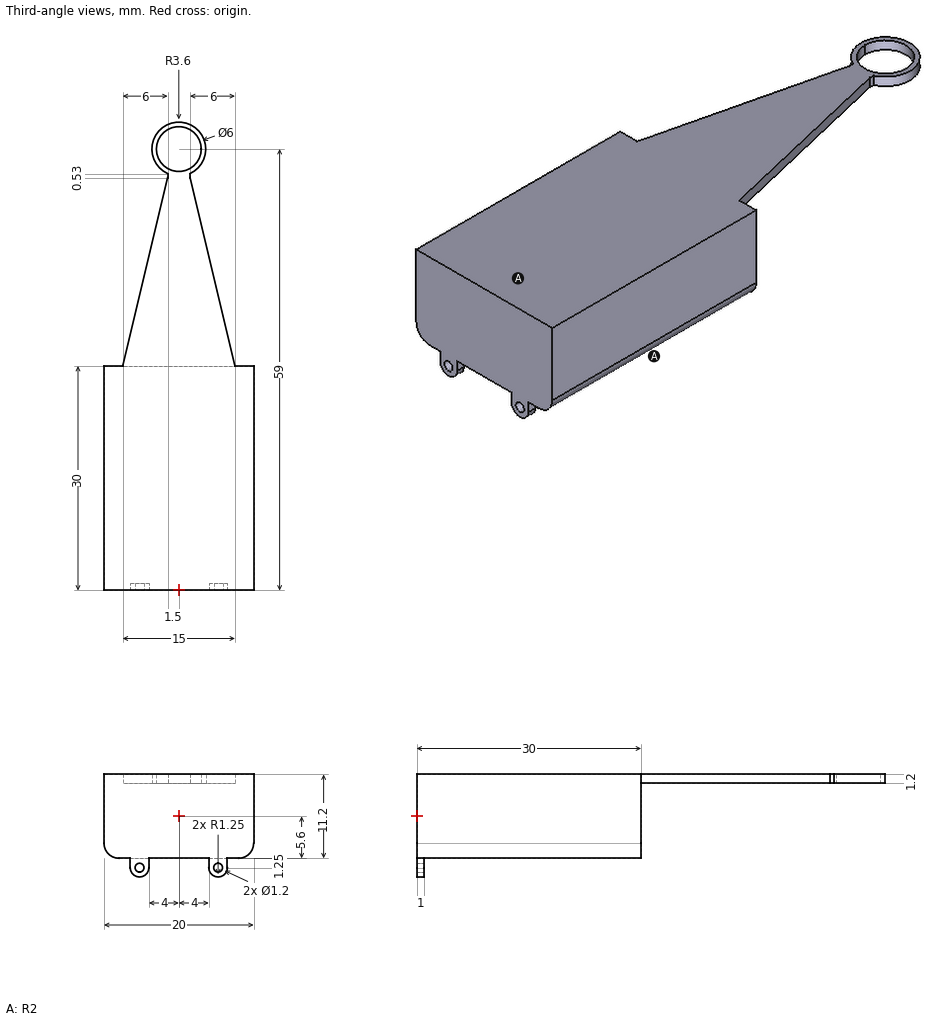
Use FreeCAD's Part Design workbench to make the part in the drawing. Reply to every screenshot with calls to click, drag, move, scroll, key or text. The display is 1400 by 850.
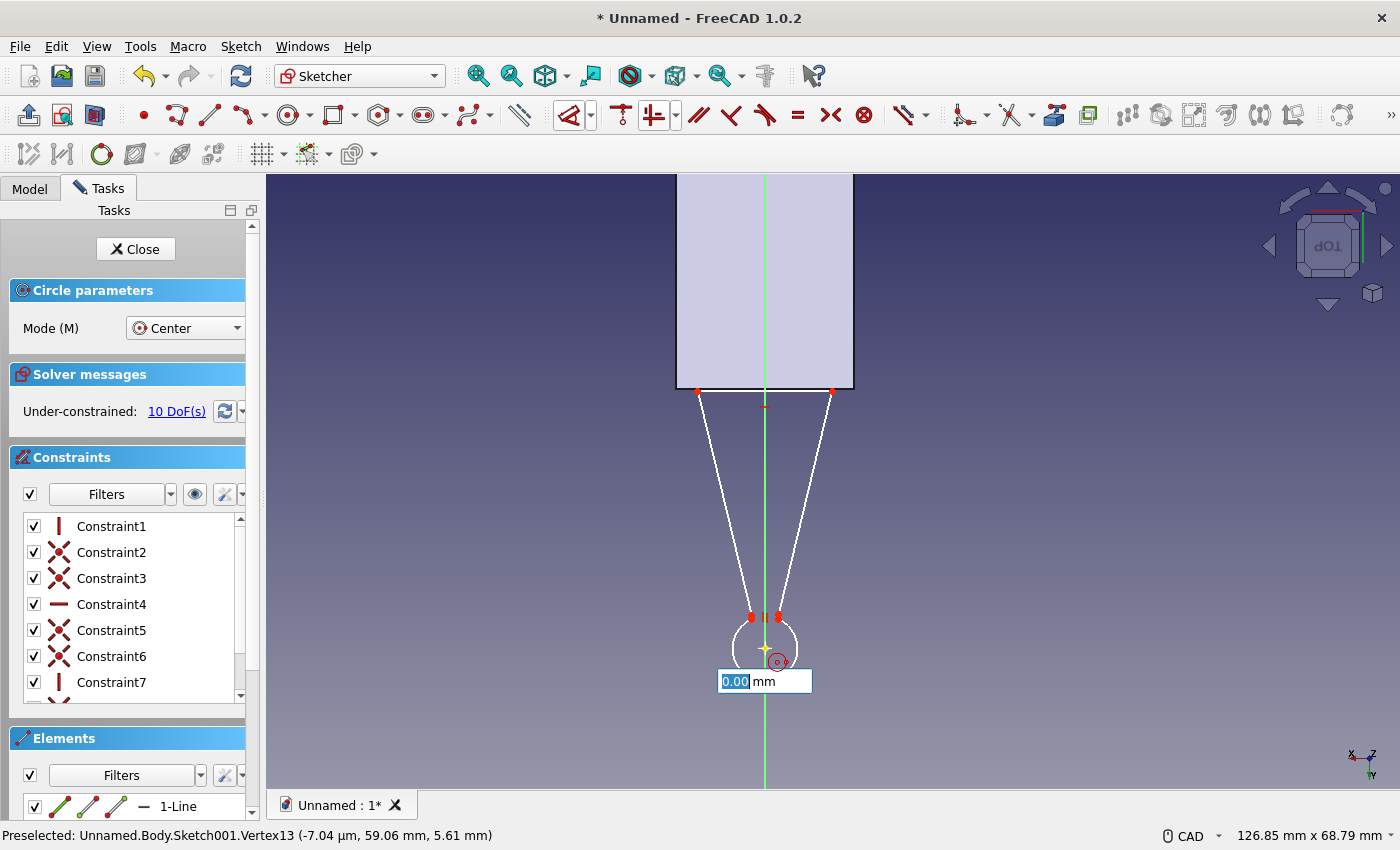
scroll(774, 623, up, 5)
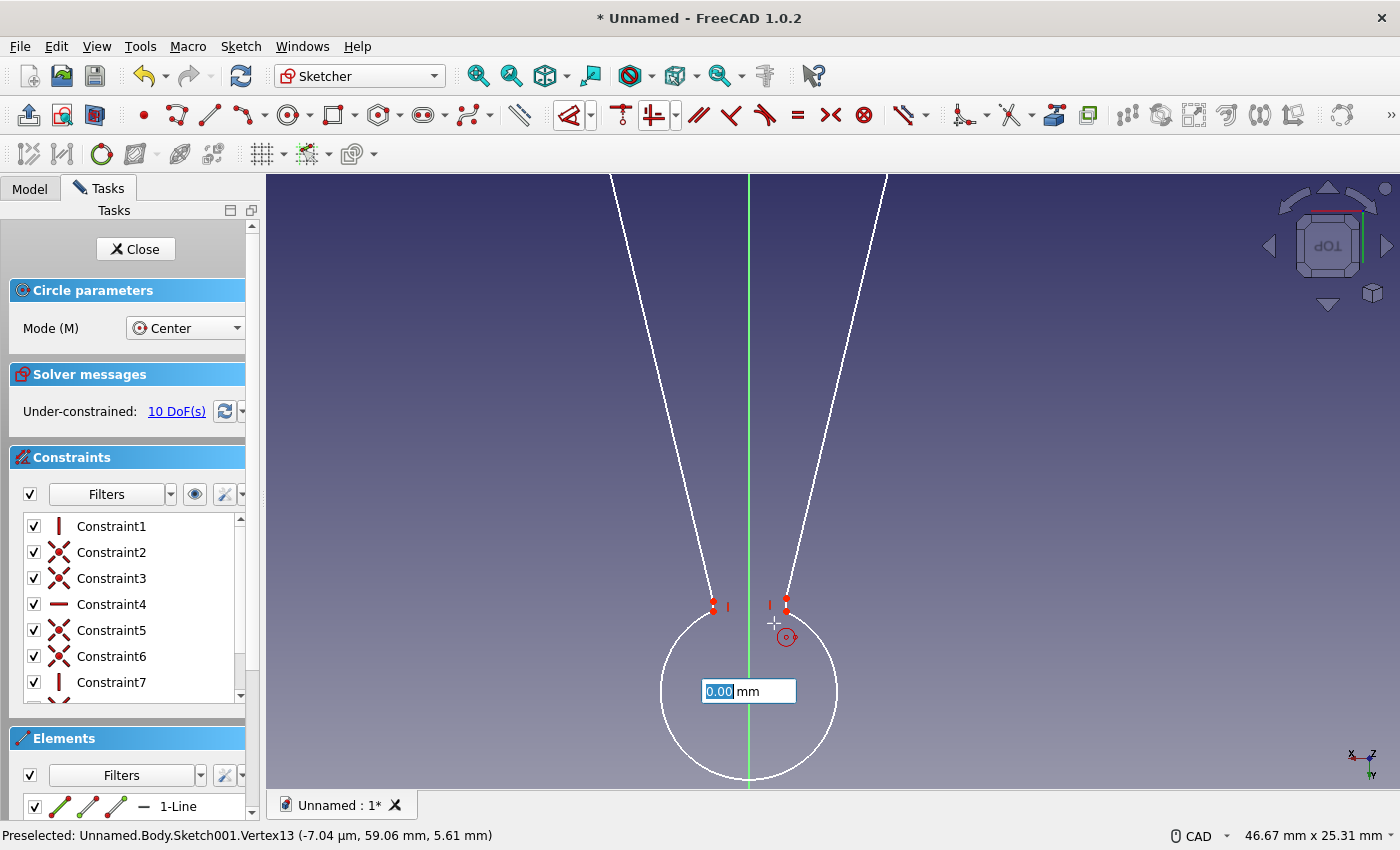
click(774, 622)
key(Escape)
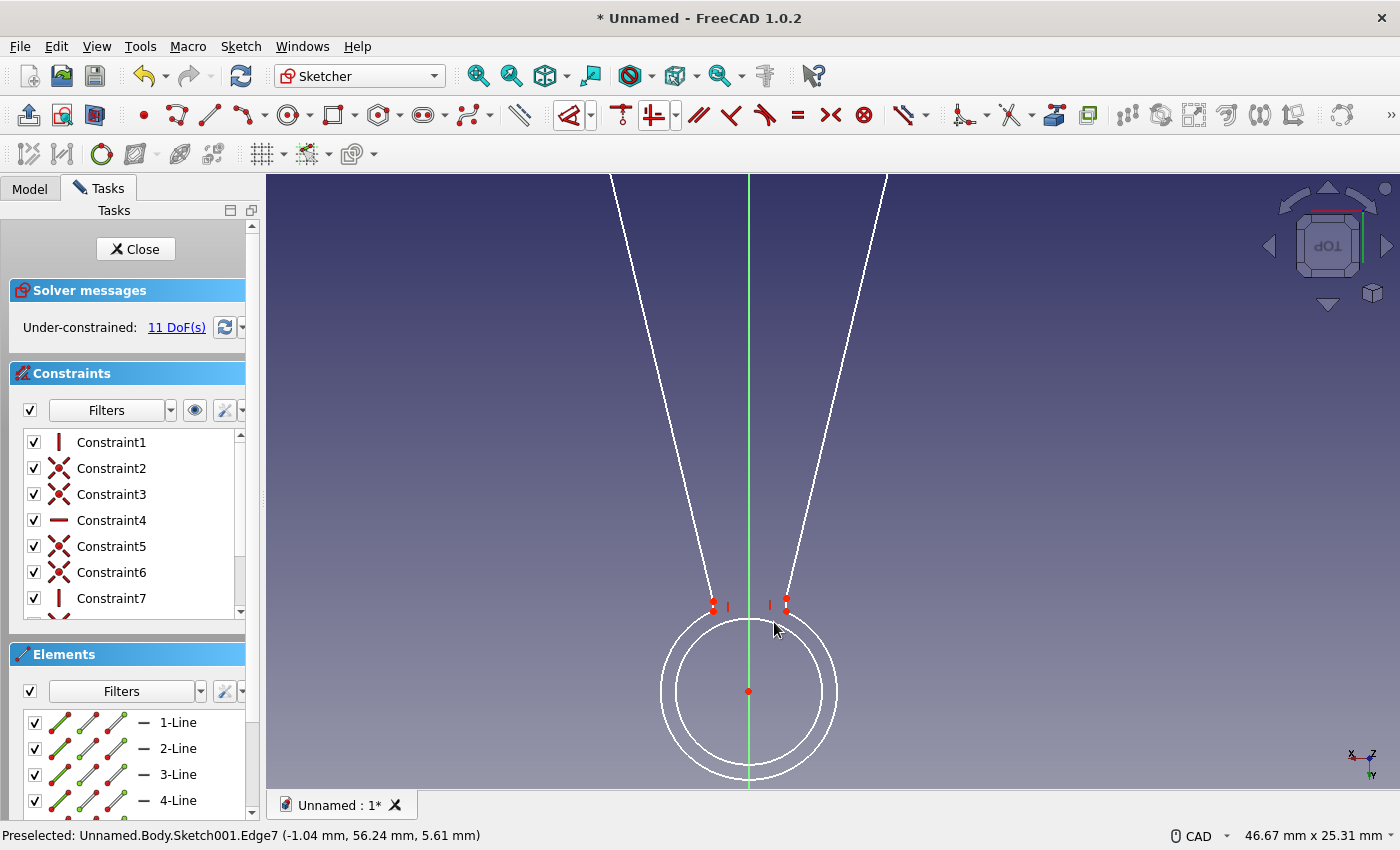
scroll(770, 634, down, 7)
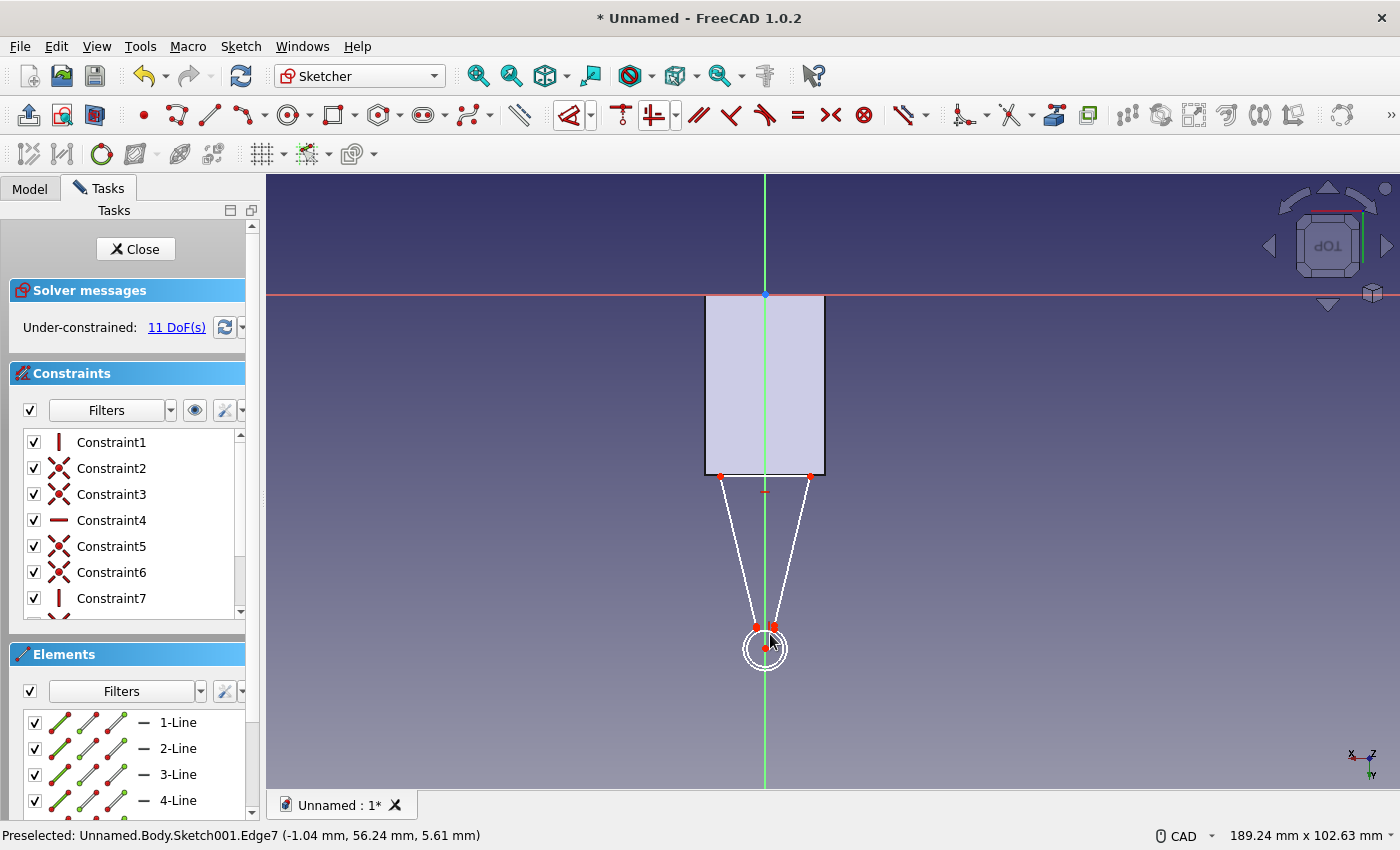
click(765, 649)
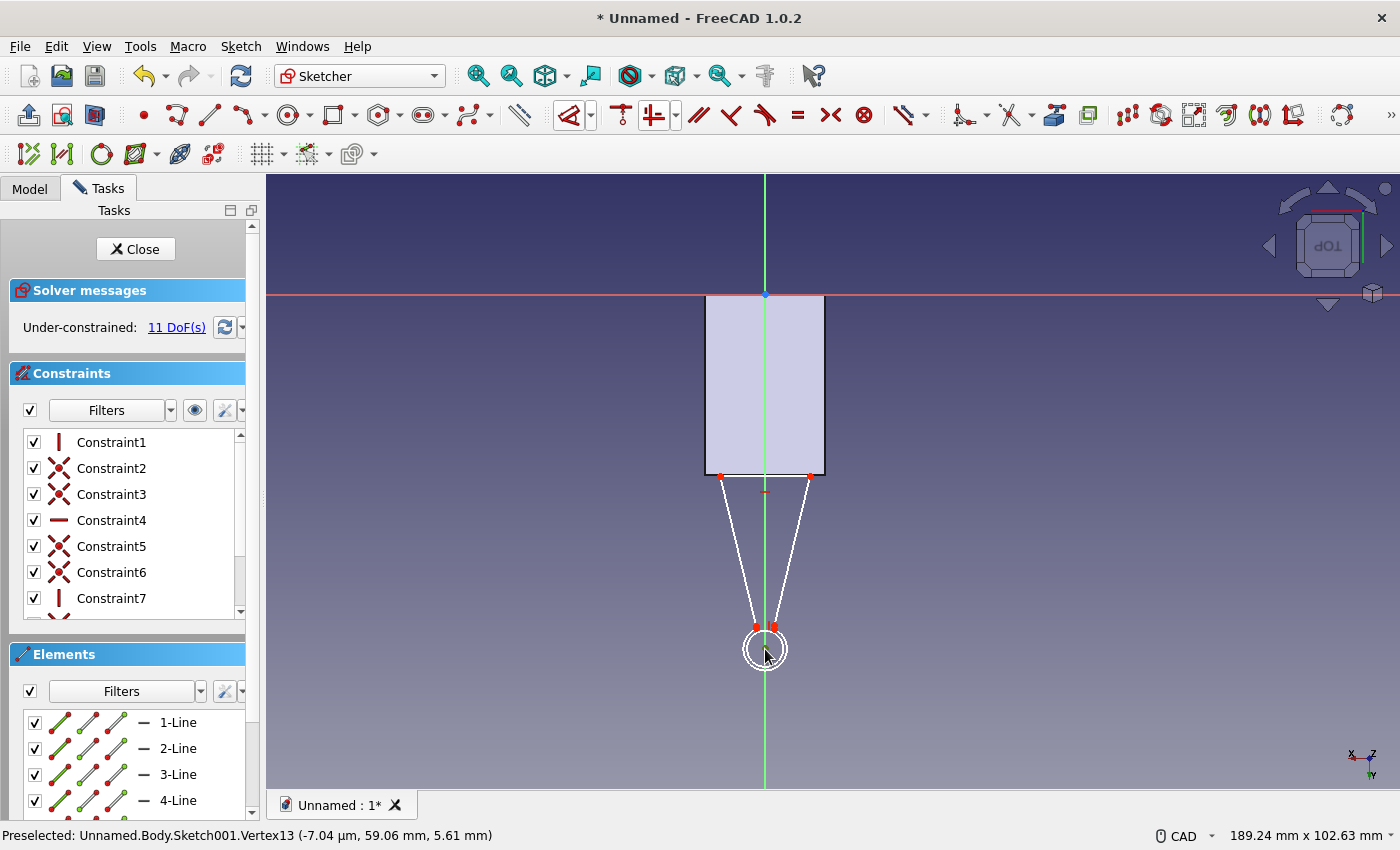
click(765, 721)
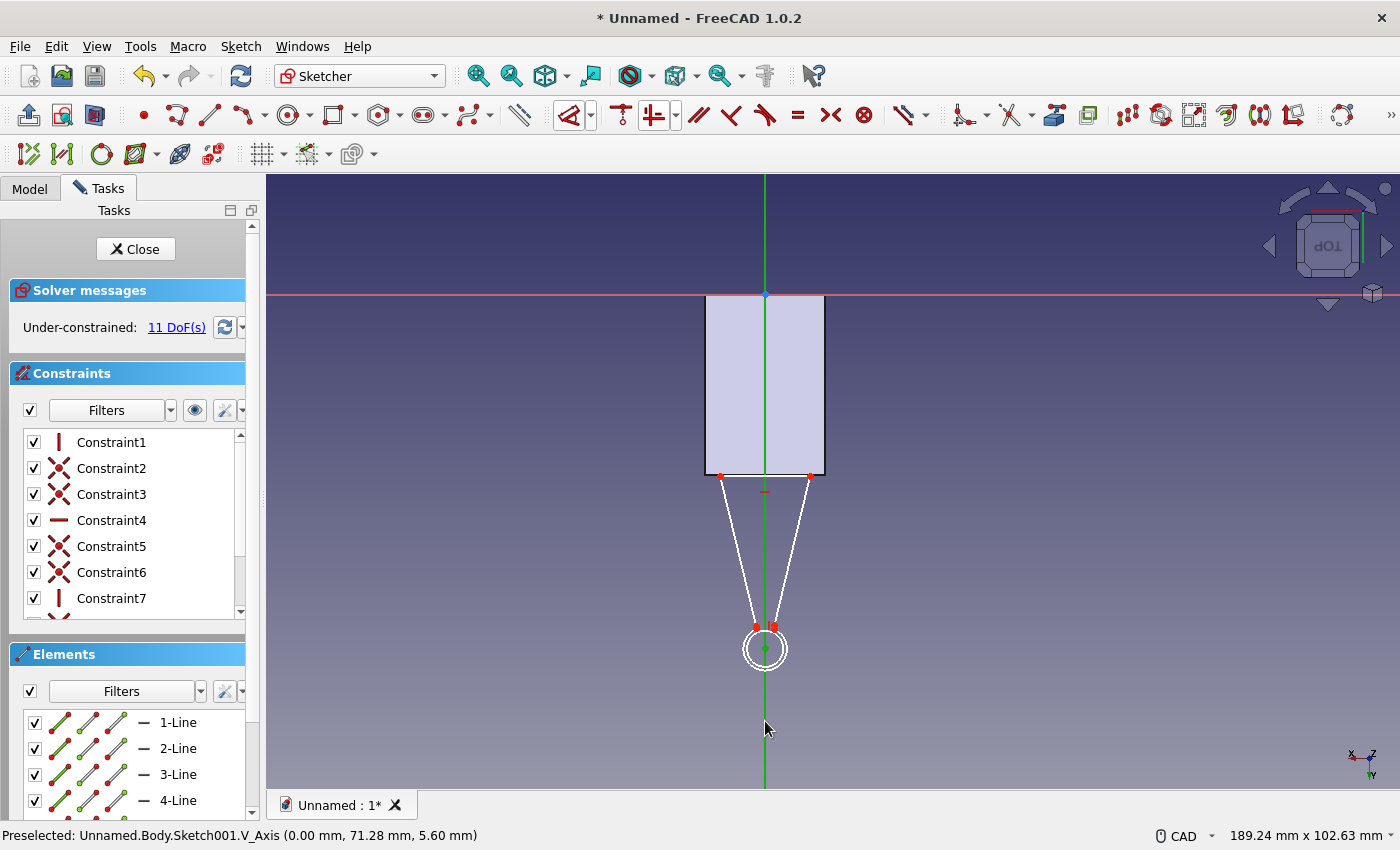
key(c)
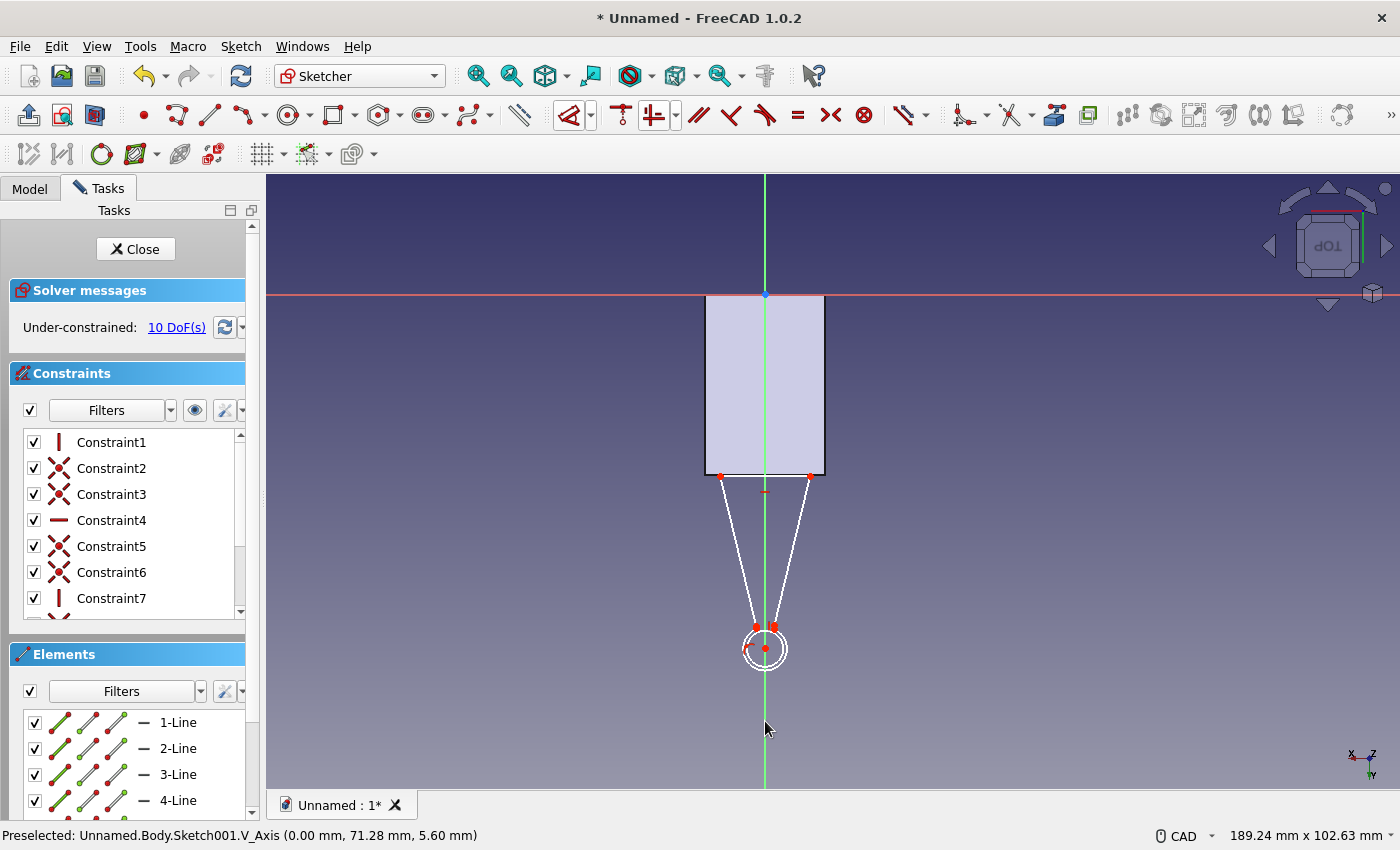
key(d)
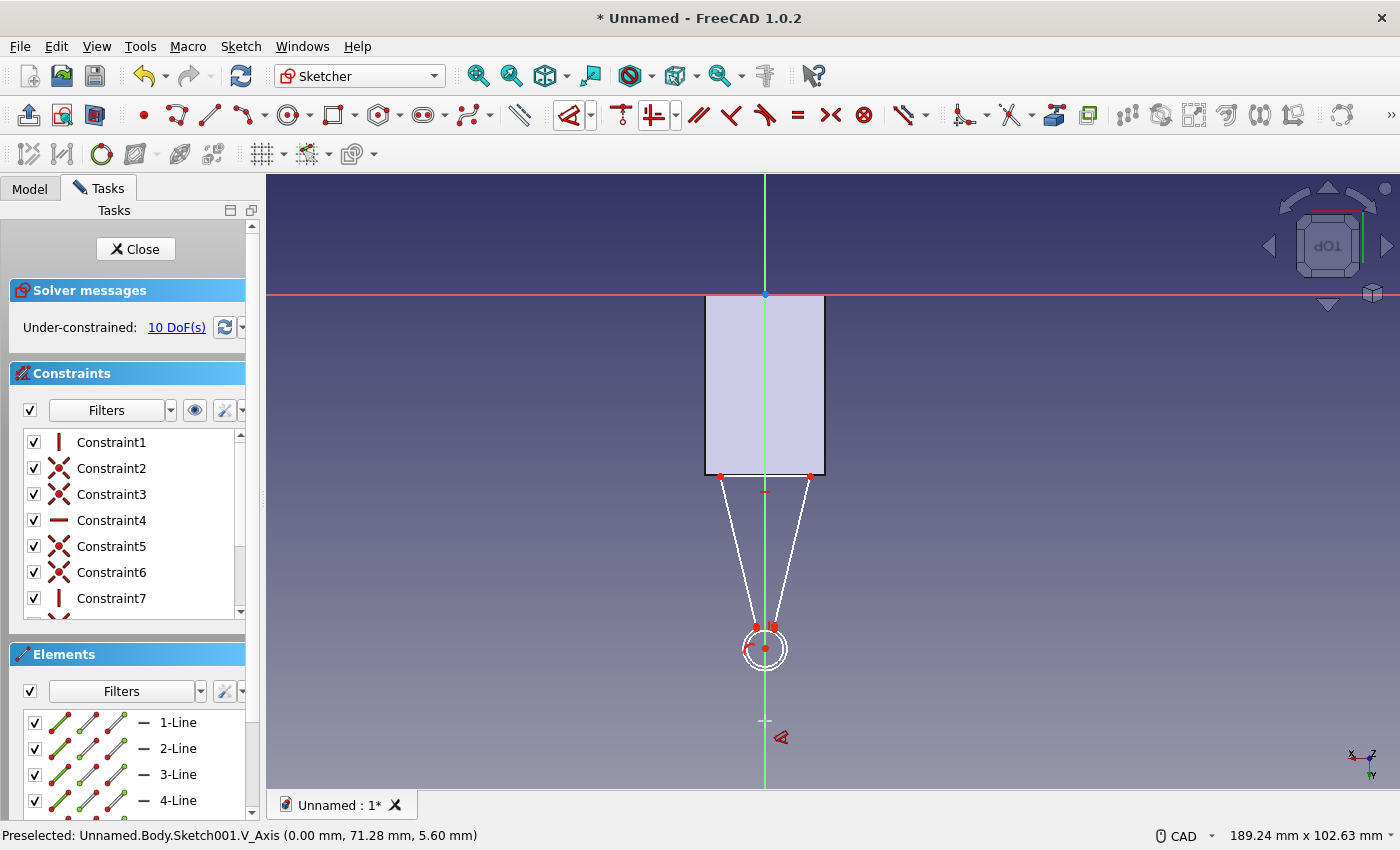
scroll(765, 671, up, 7)